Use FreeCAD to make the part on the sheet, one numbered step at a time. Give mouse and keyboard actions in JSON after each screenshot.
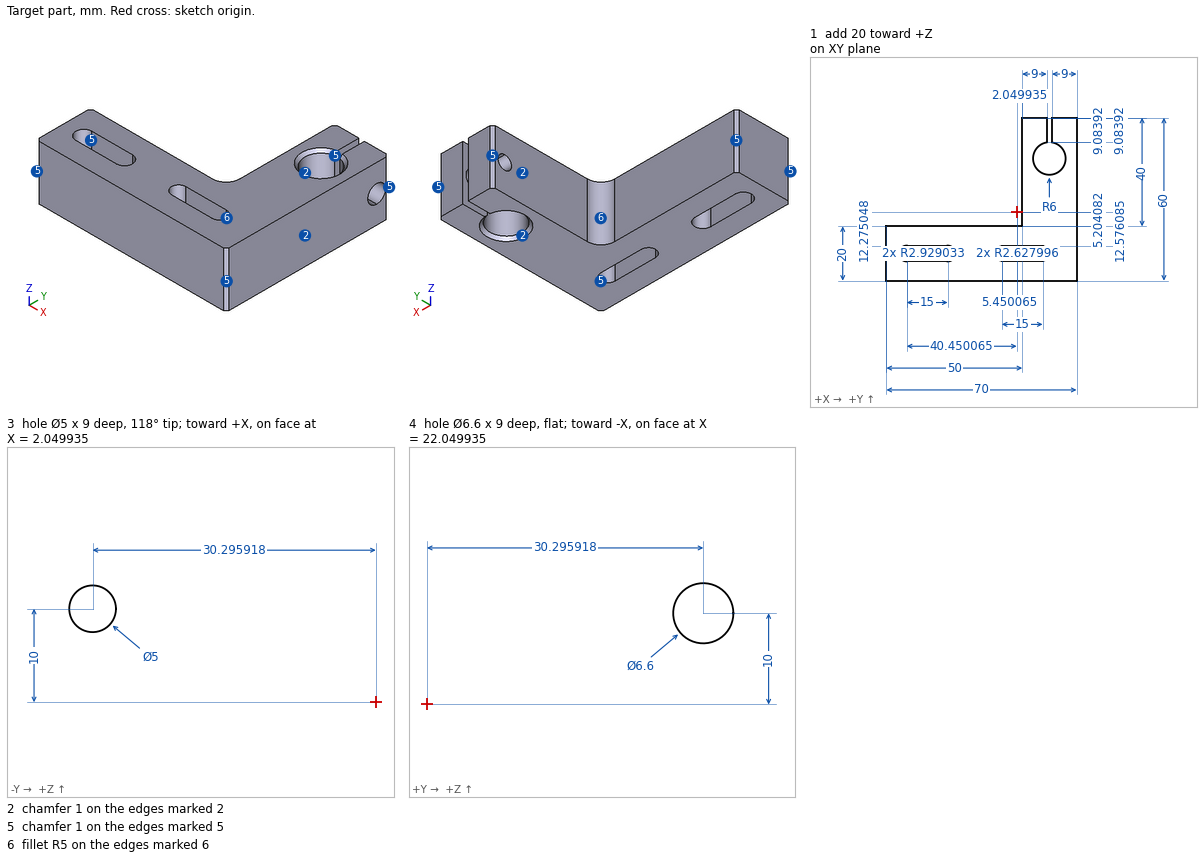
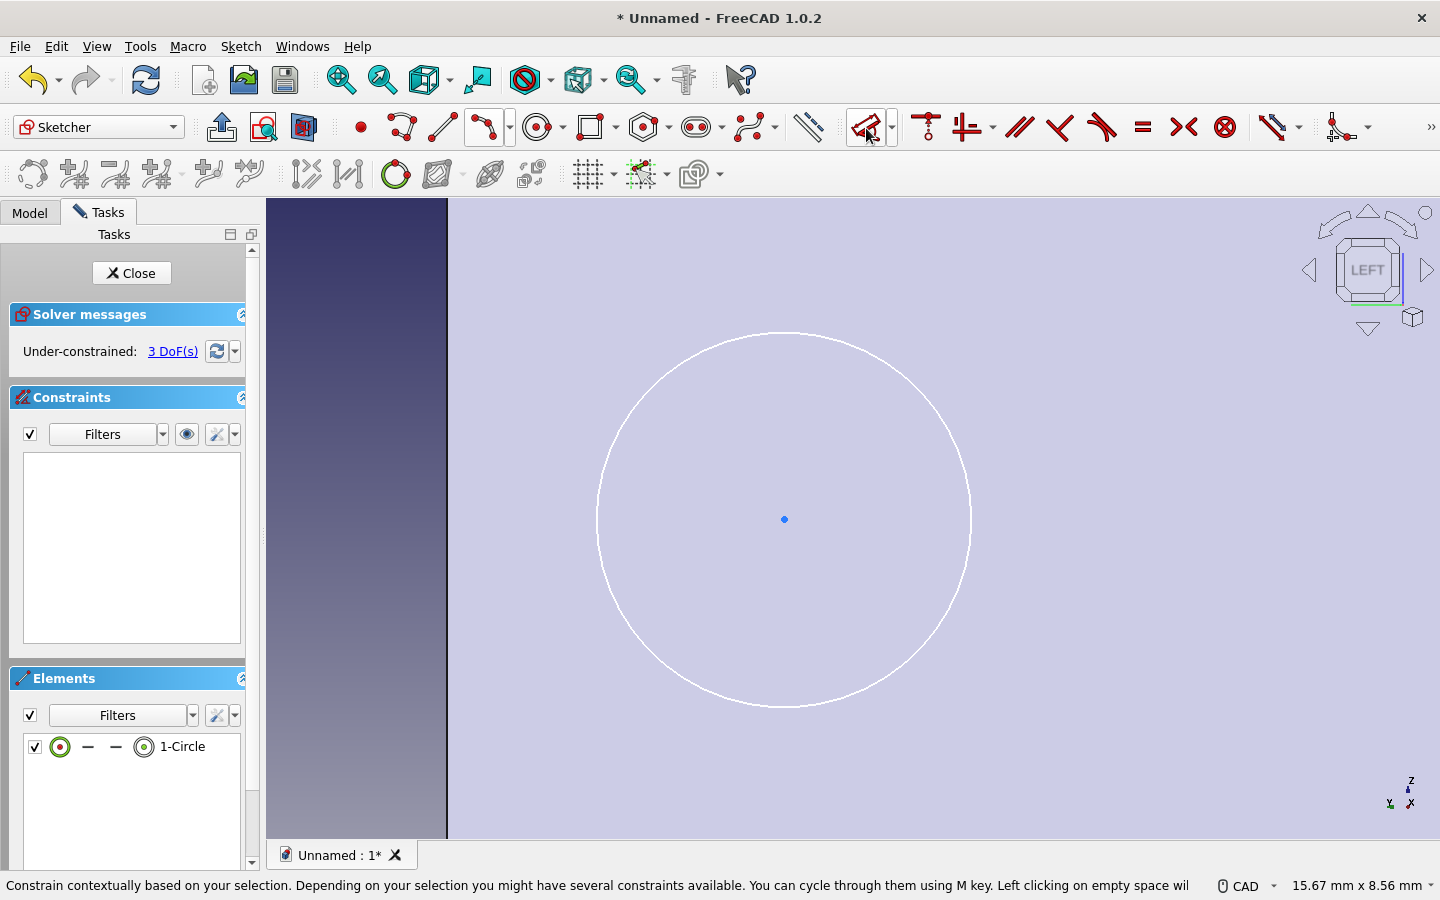
{"action": "left_click", "coordinate": [916, 387]}
{"action": "left_click", "coordinate": [939, 364]}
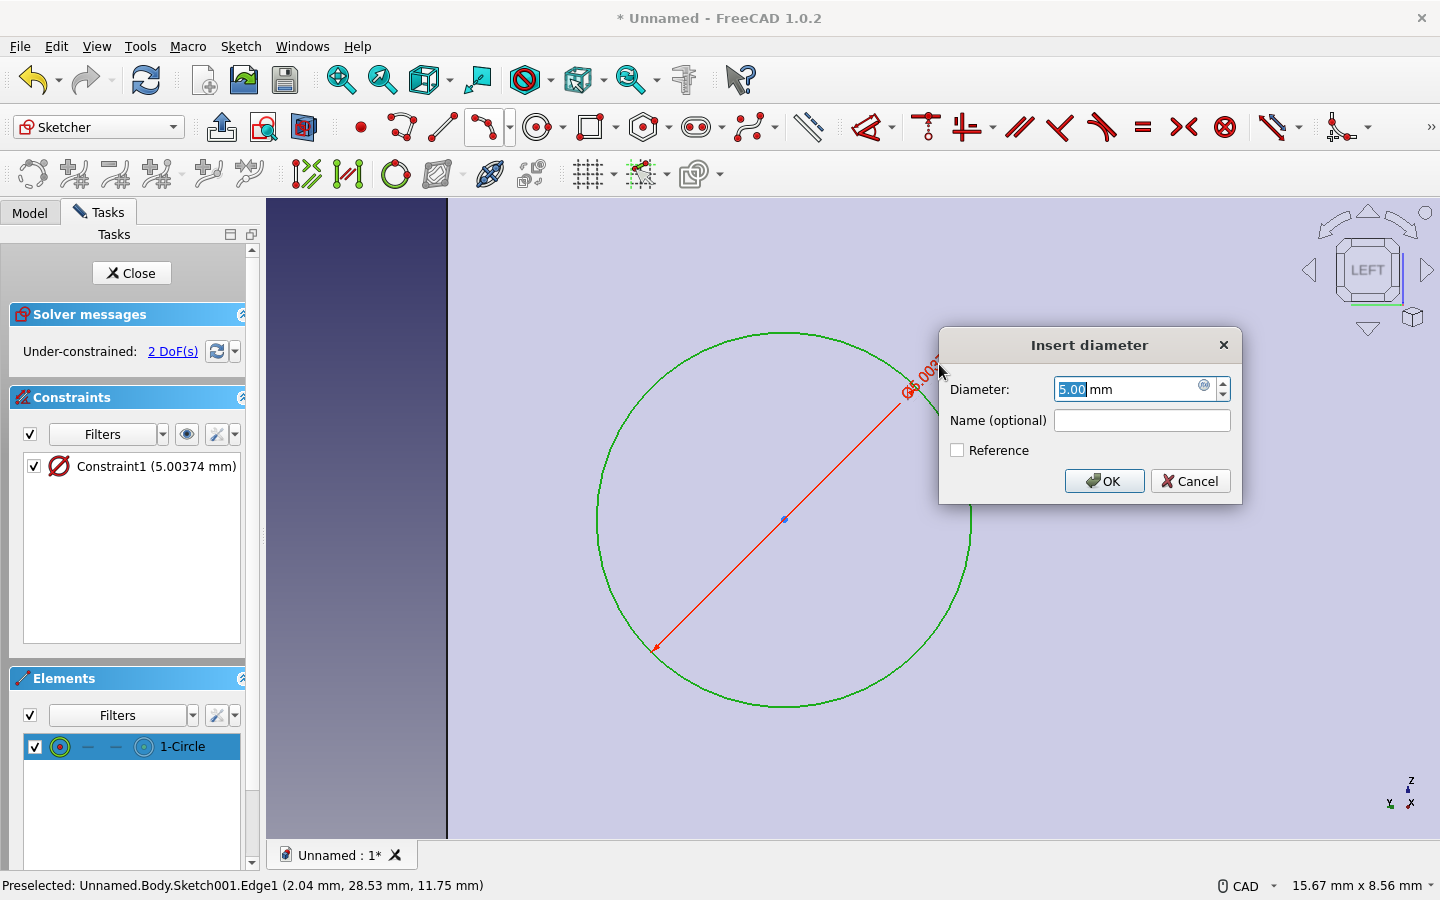
{"action": "type", "text": "5"}
{"action": "key", "text": "Return"}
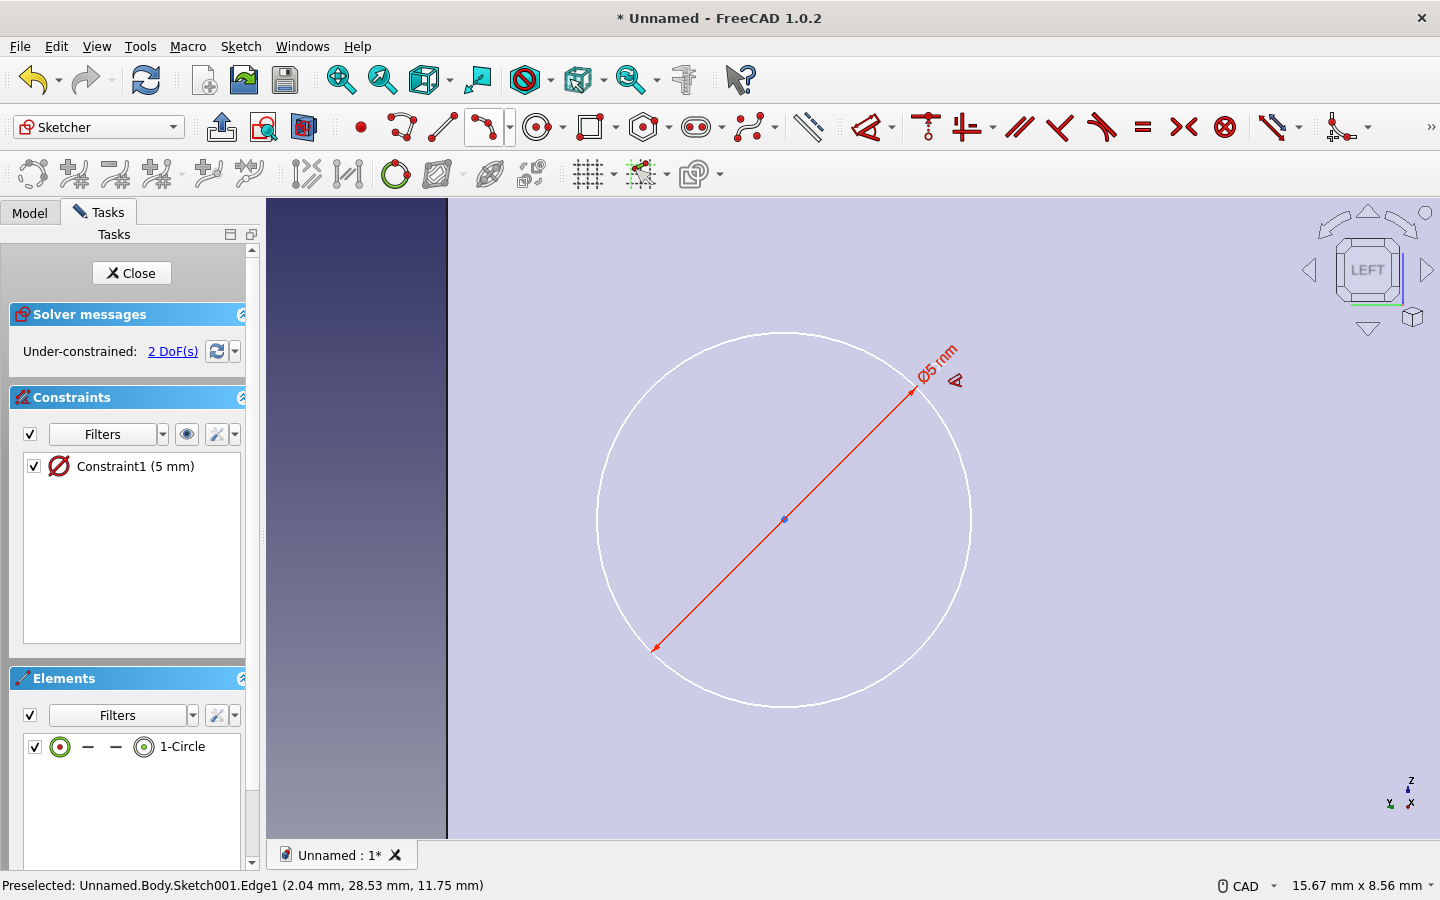
{"action": "left_click", "coordinate": [784, 520]}
{"action": "left_click", "coordinate": [750, 665]}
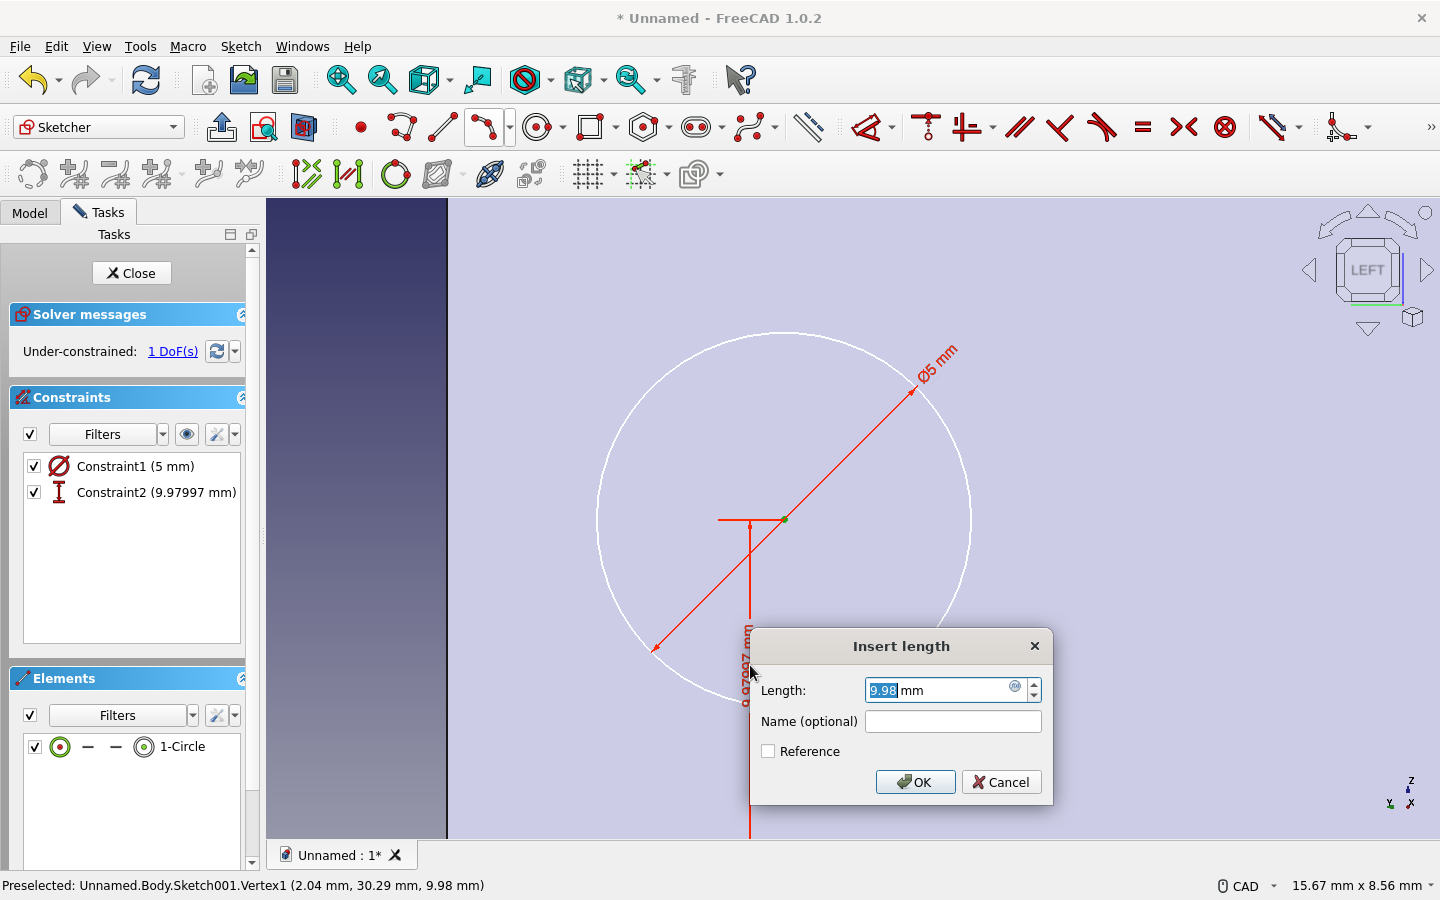
{"action": "type", "text": "10"}
{"action": "key", "text": "Return"}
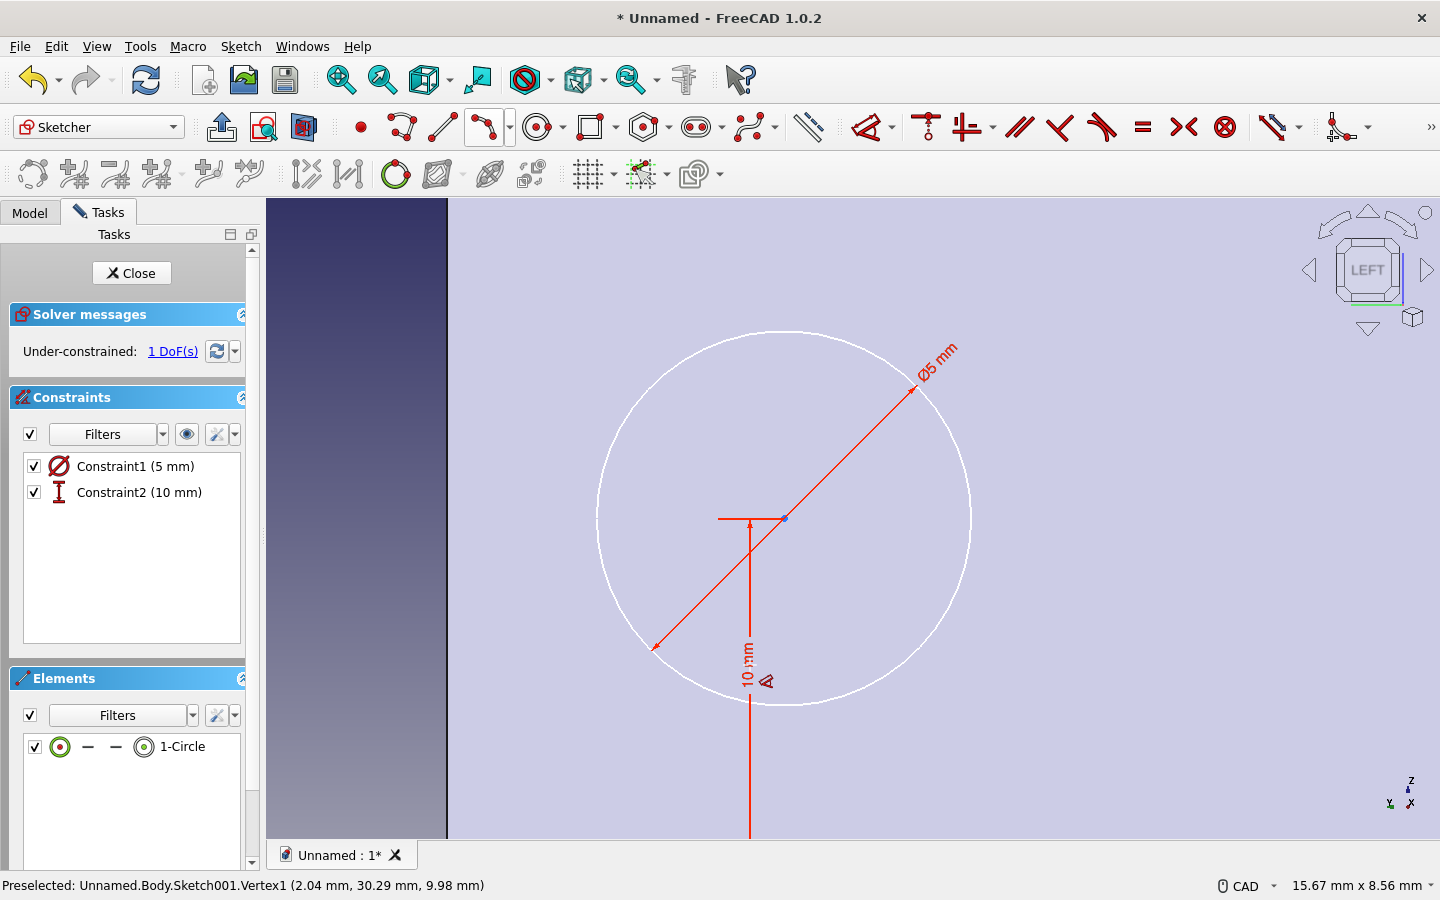
{"action": "left_click", "coordinate": [784, 519]}
{"action": "left_click", "coordinate": [1030, 485]}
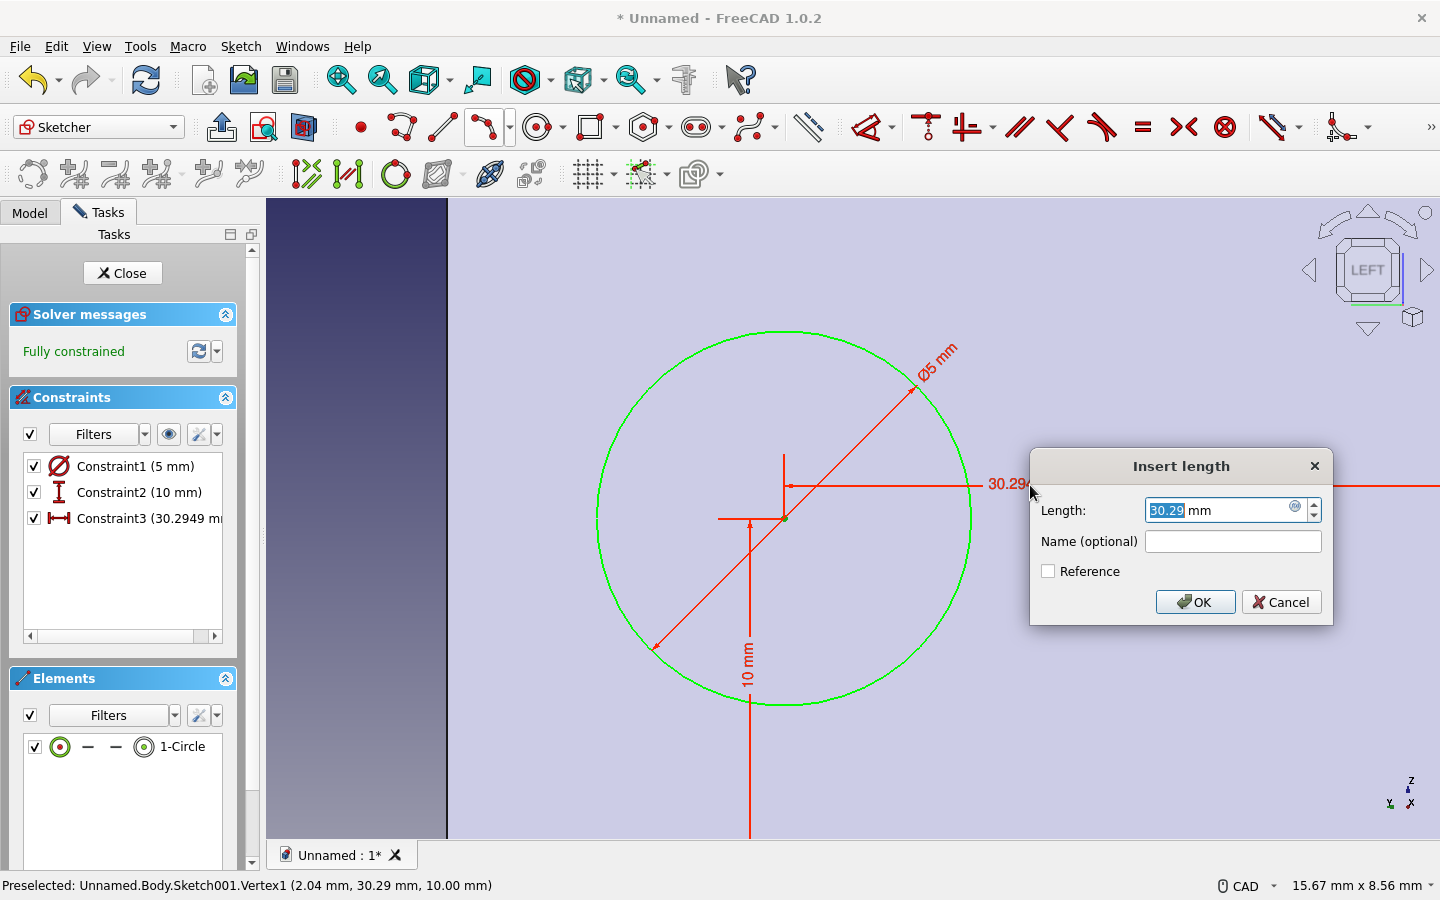
{"action": "type", "text": "30.295918"}
{"action": "key", "text": "Return"}
{"action": "key", "text": "Escape"}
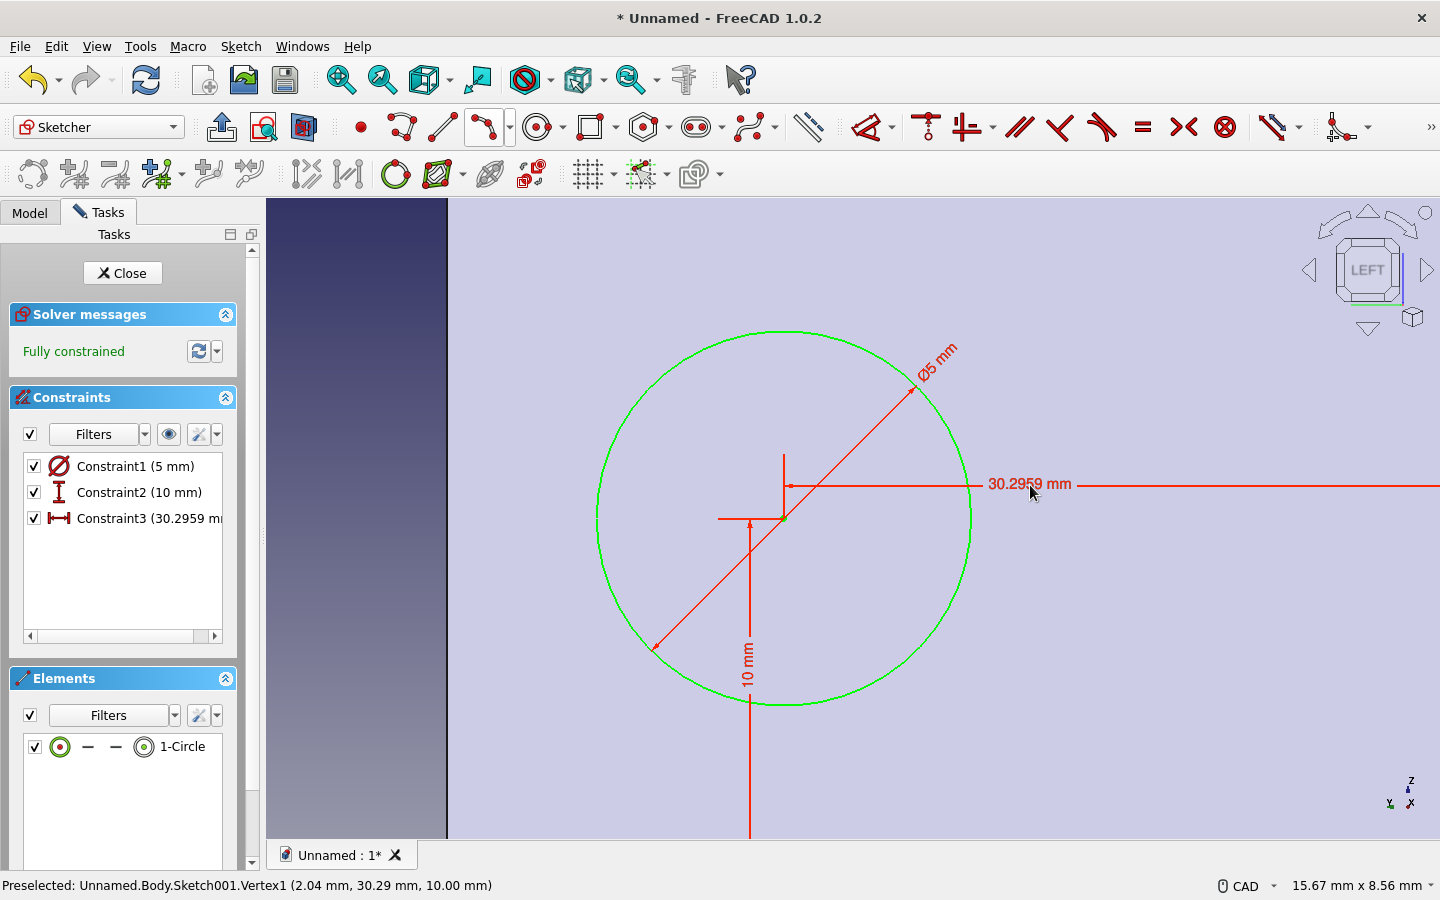
{"action": "left_click", "coordinate": [123, 273]}